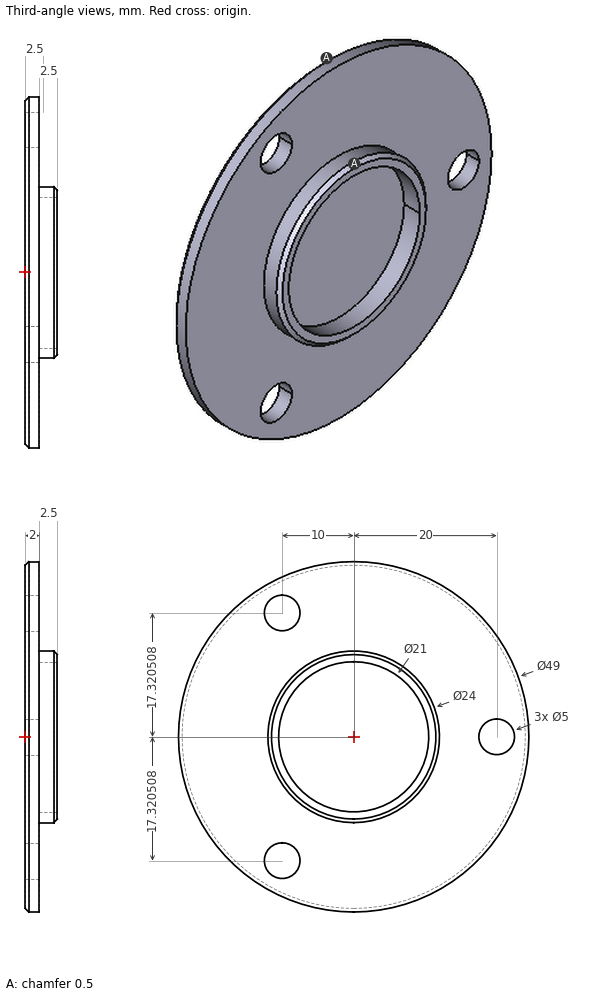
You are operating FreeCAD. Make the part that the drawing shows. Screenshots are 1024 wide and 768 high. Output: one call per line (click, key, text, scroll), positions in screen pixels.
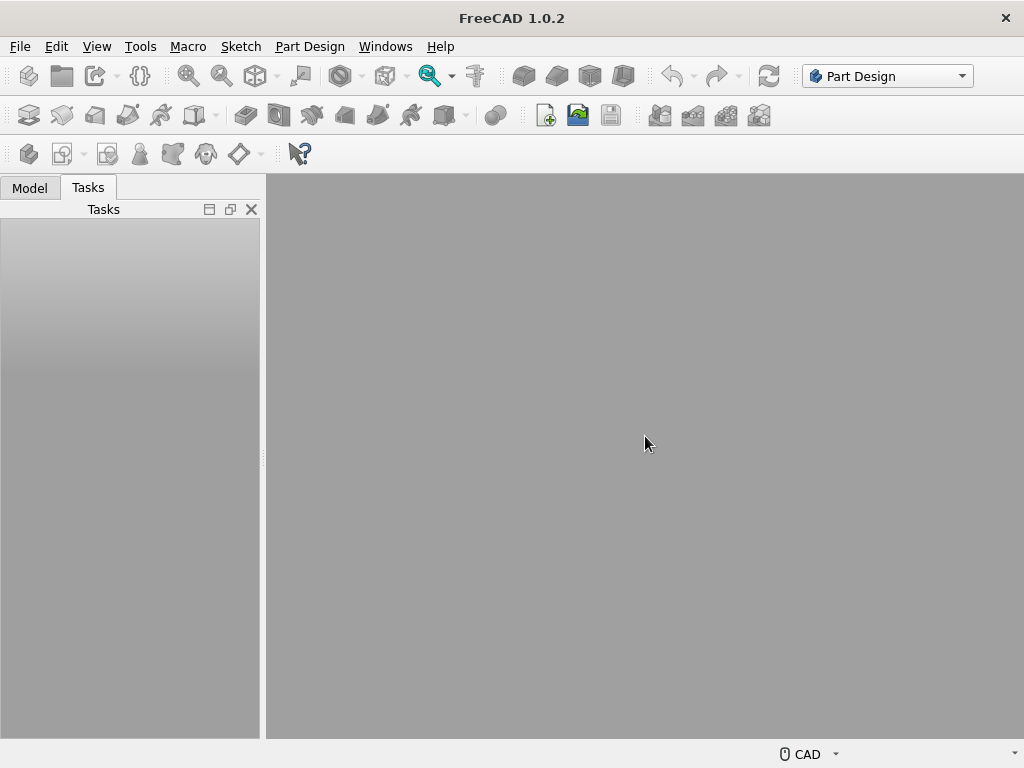
click(545, 116)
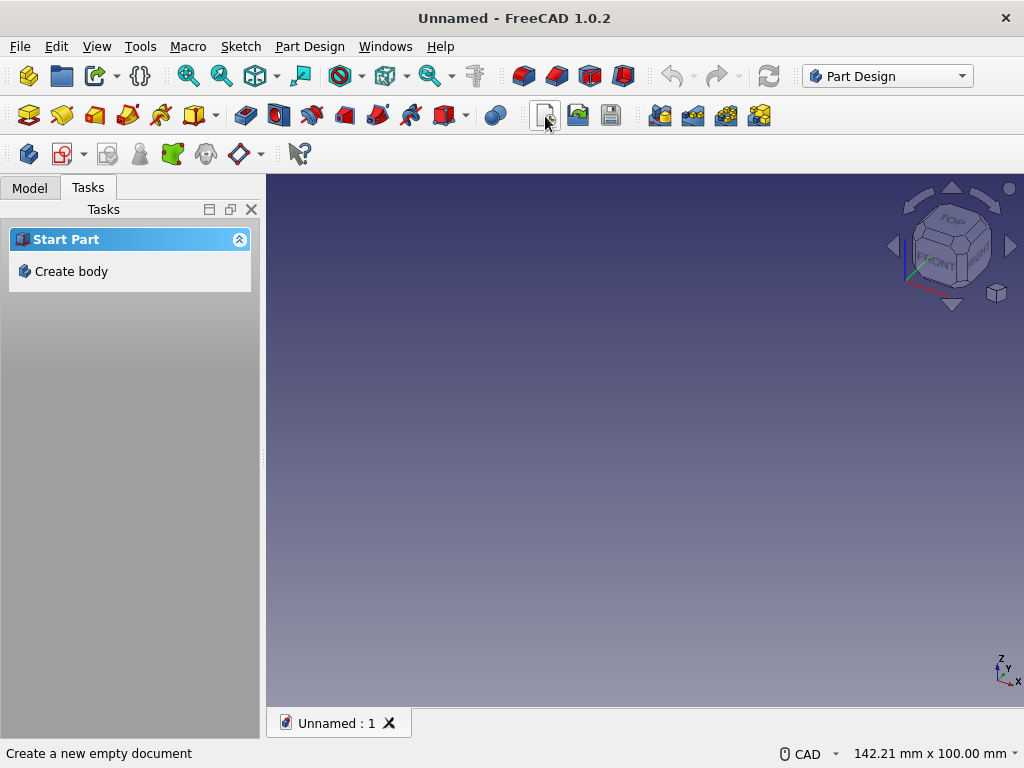
click(62, 154)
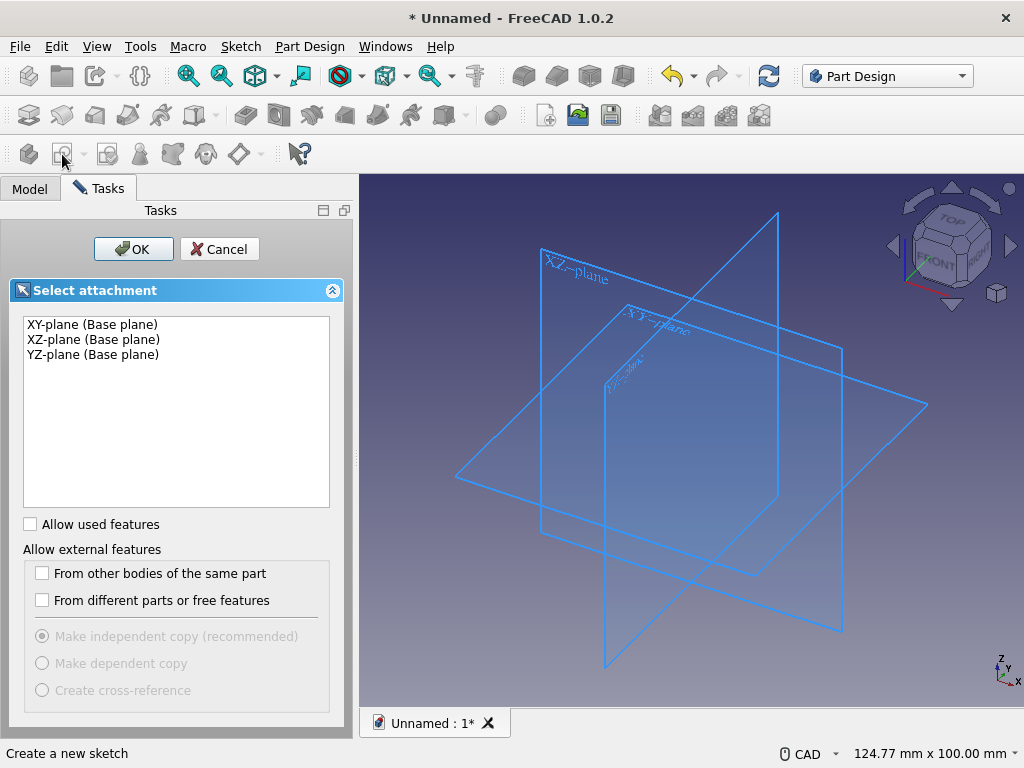
click(84, 354)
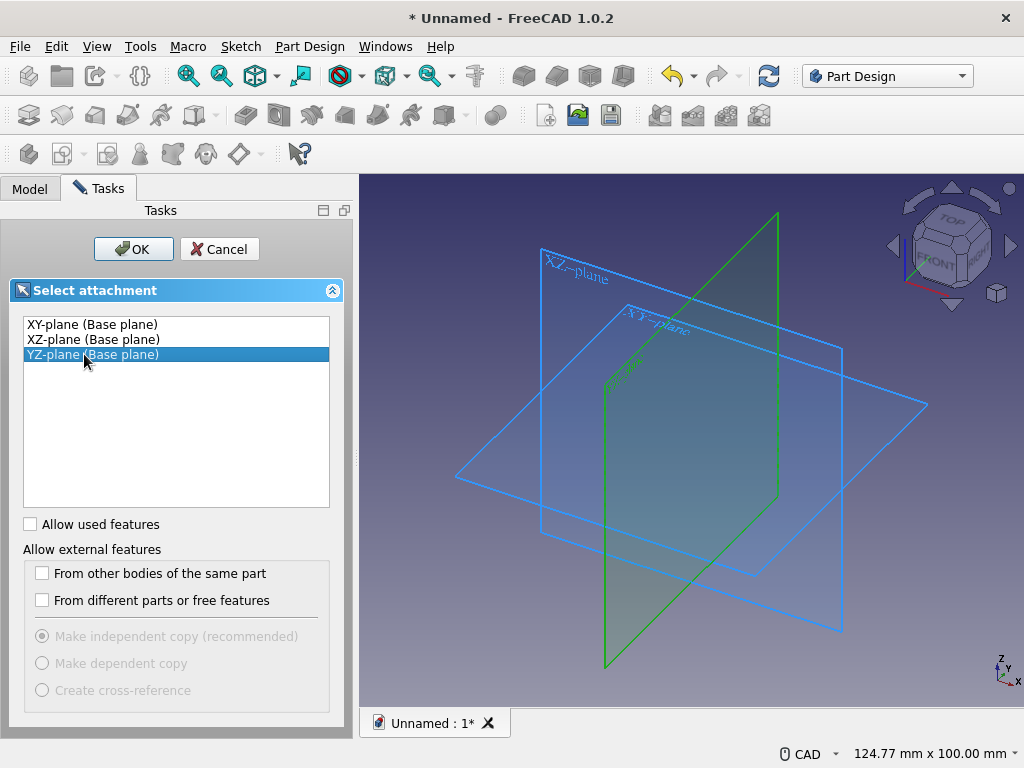
click(134, 249)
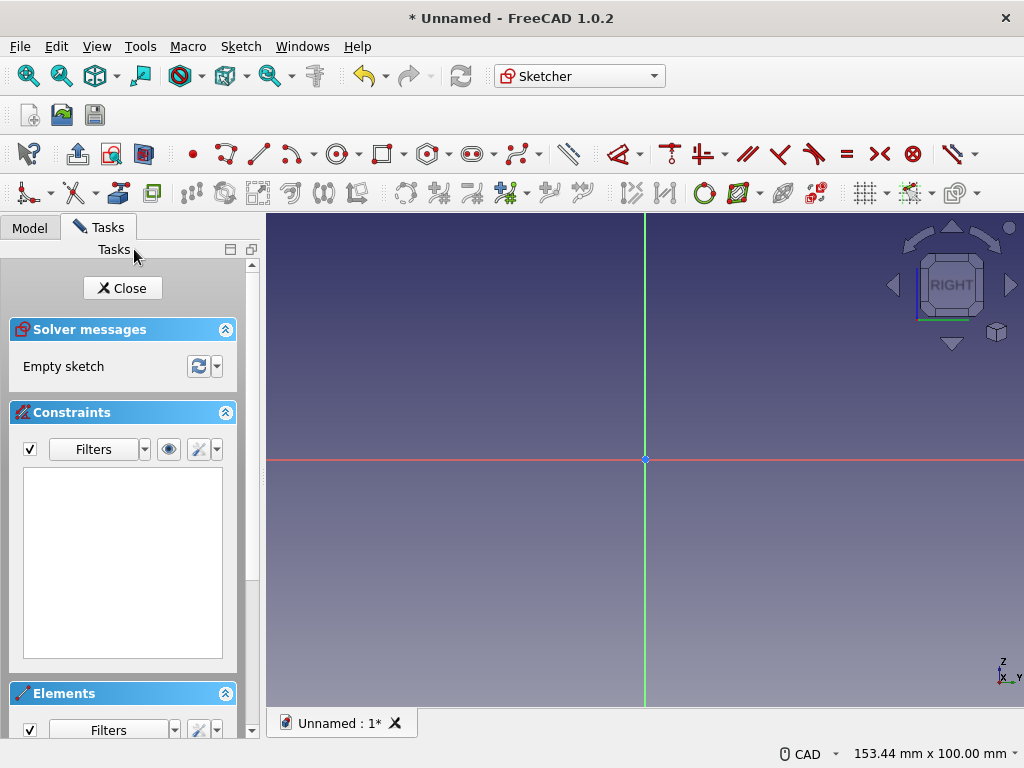
click(336, 154)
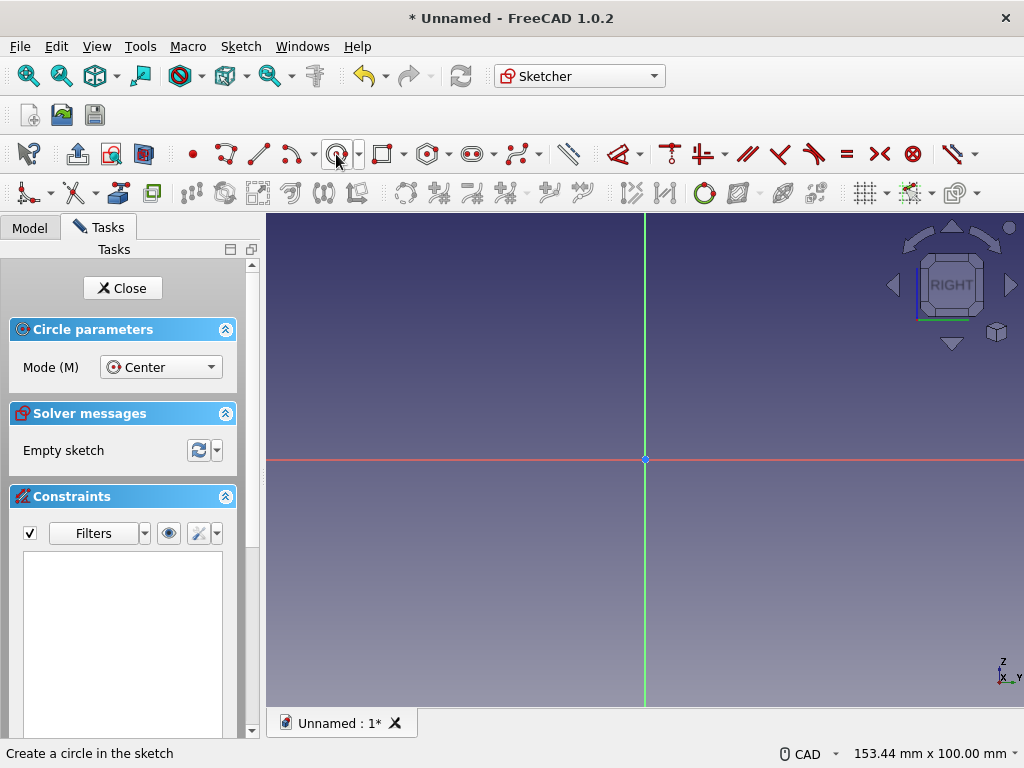
click(645, 460)
click(731, 374)
key(Escape)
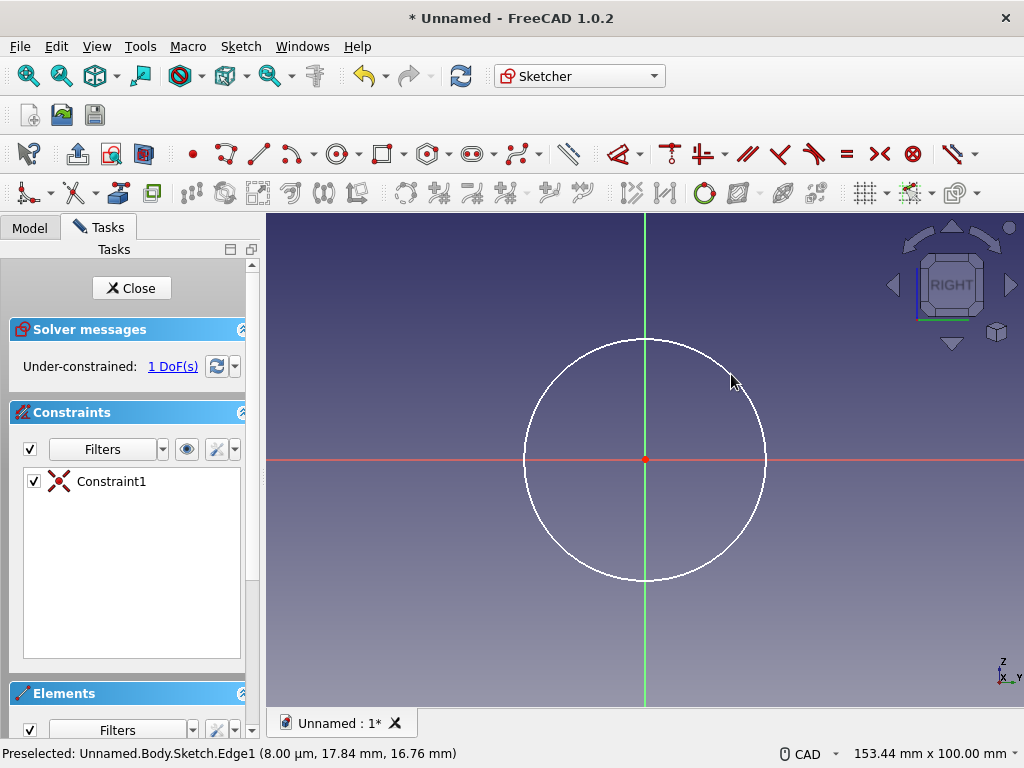
click(618, 154)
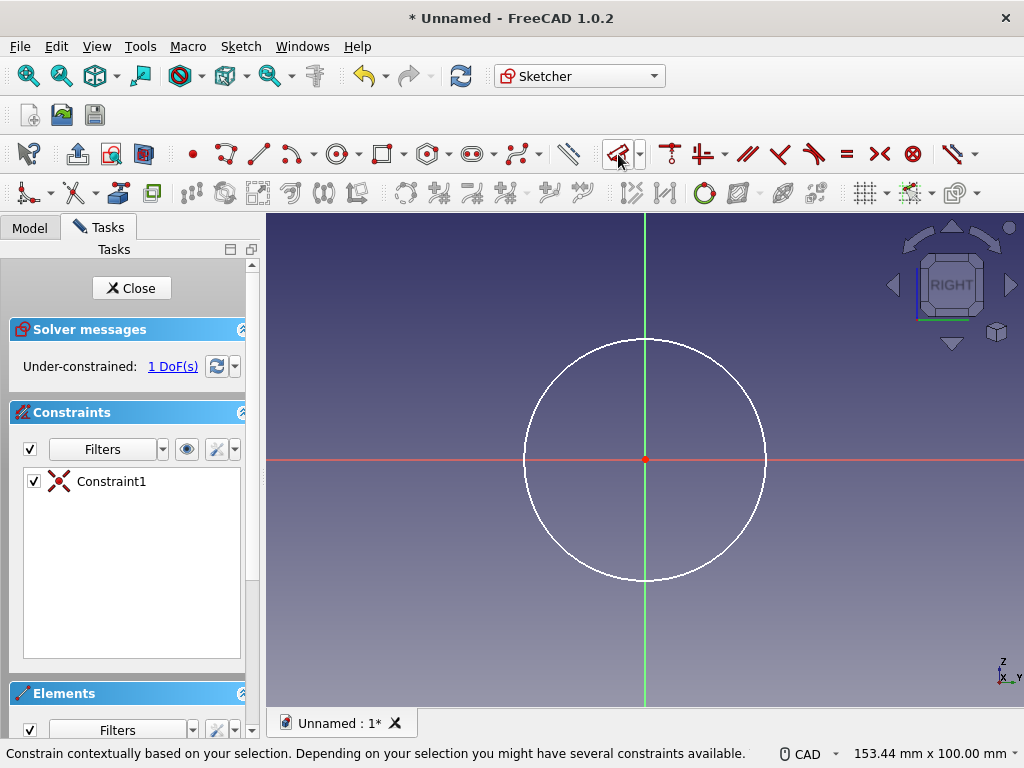
click(730, 374)
click(752, 351)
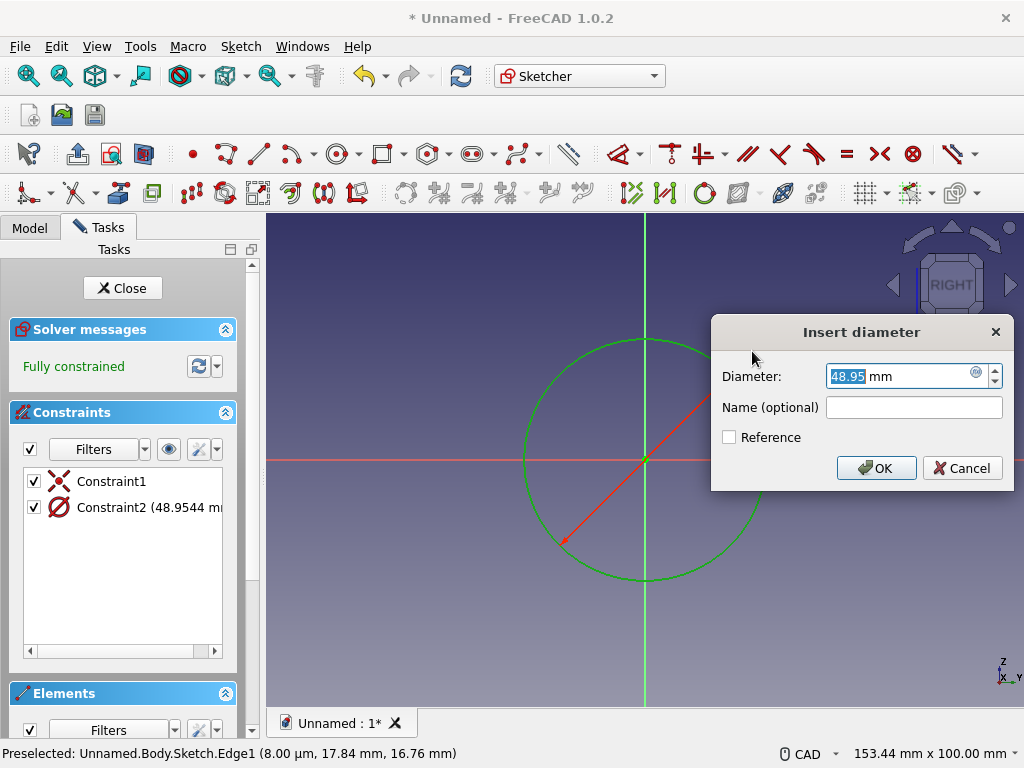
text(49)
key(Return)
key(Escape)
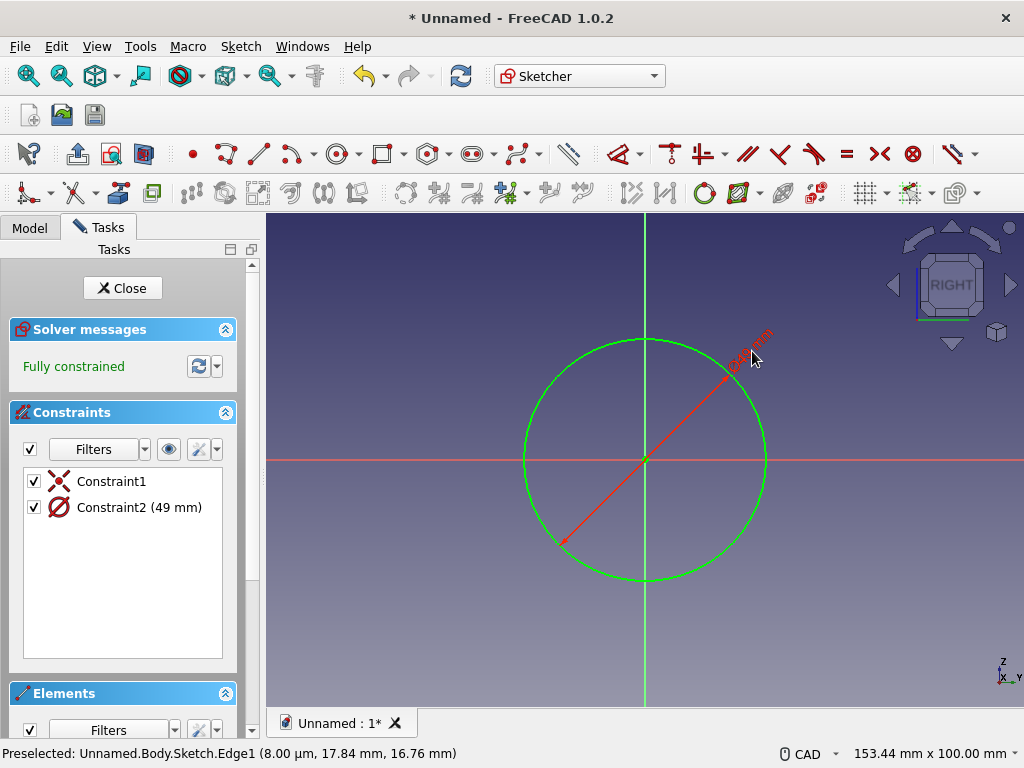
click(123, 288)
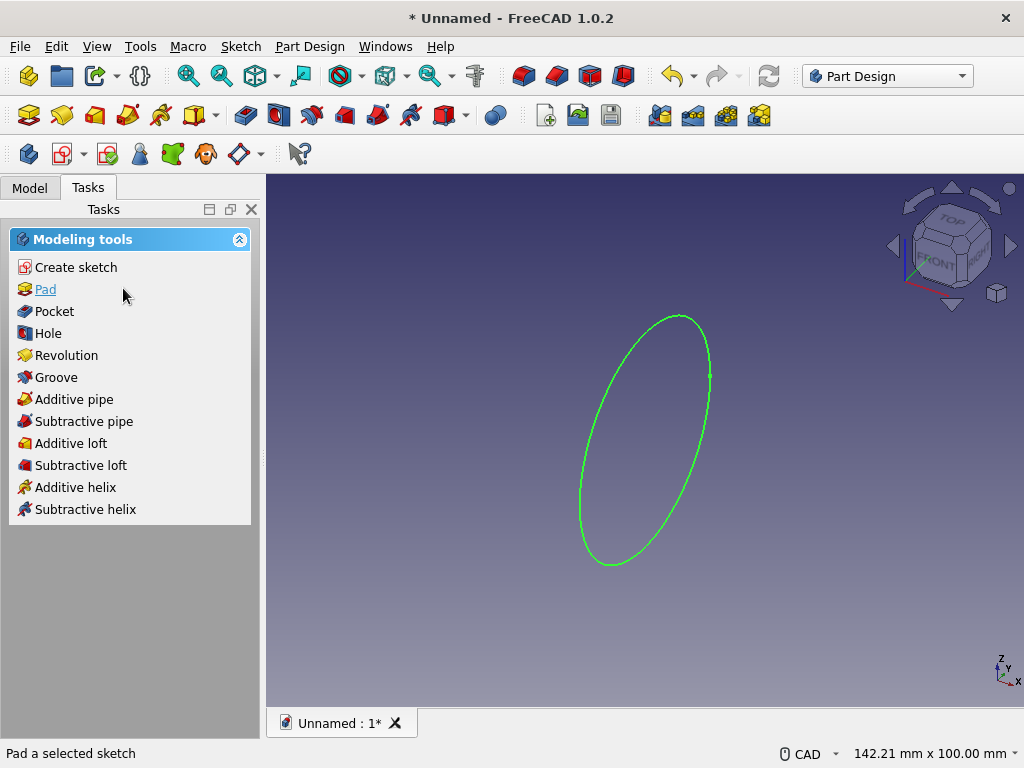
click(29, 116)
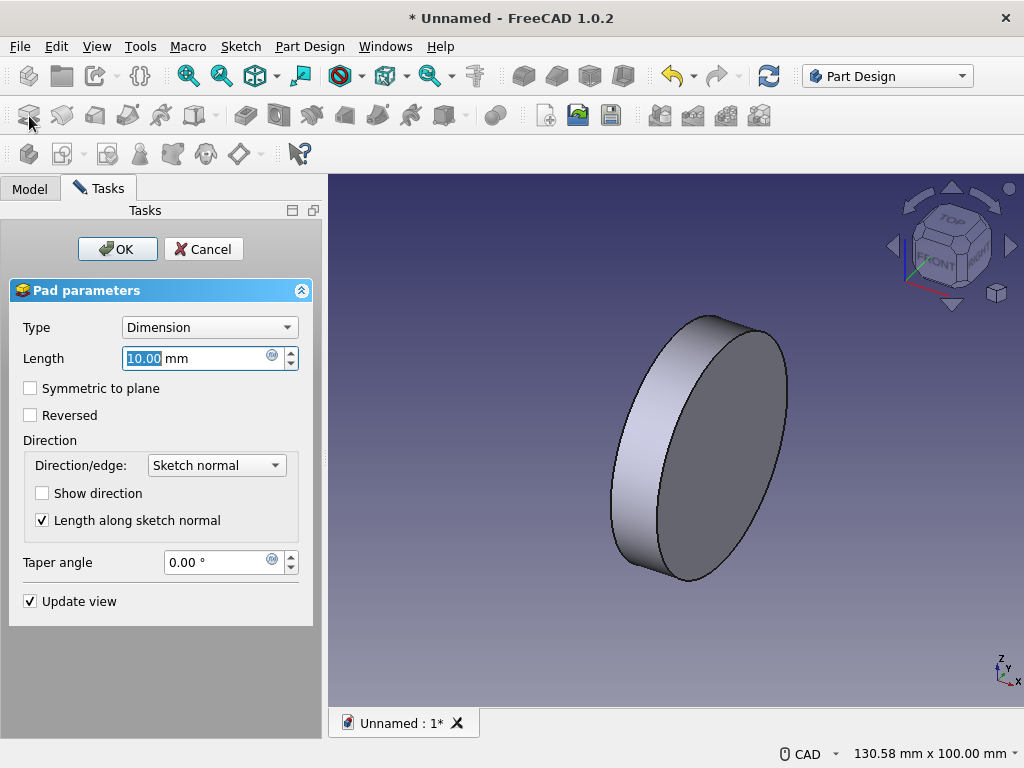
text(2)
key(Tab)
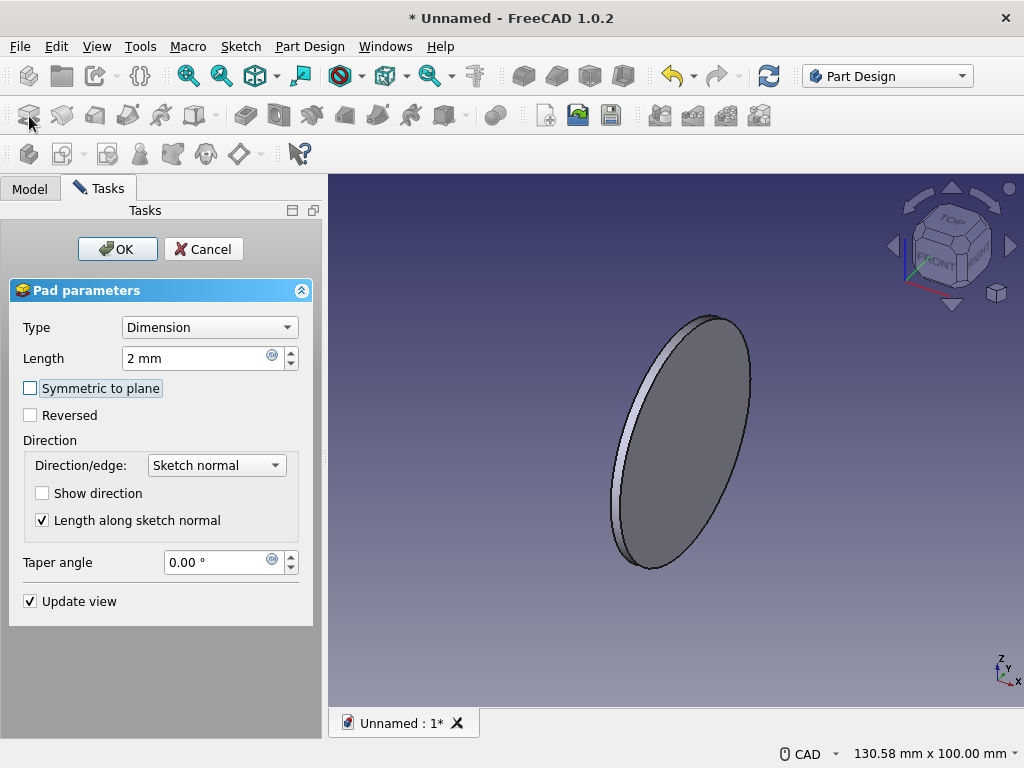
click(118, 249)